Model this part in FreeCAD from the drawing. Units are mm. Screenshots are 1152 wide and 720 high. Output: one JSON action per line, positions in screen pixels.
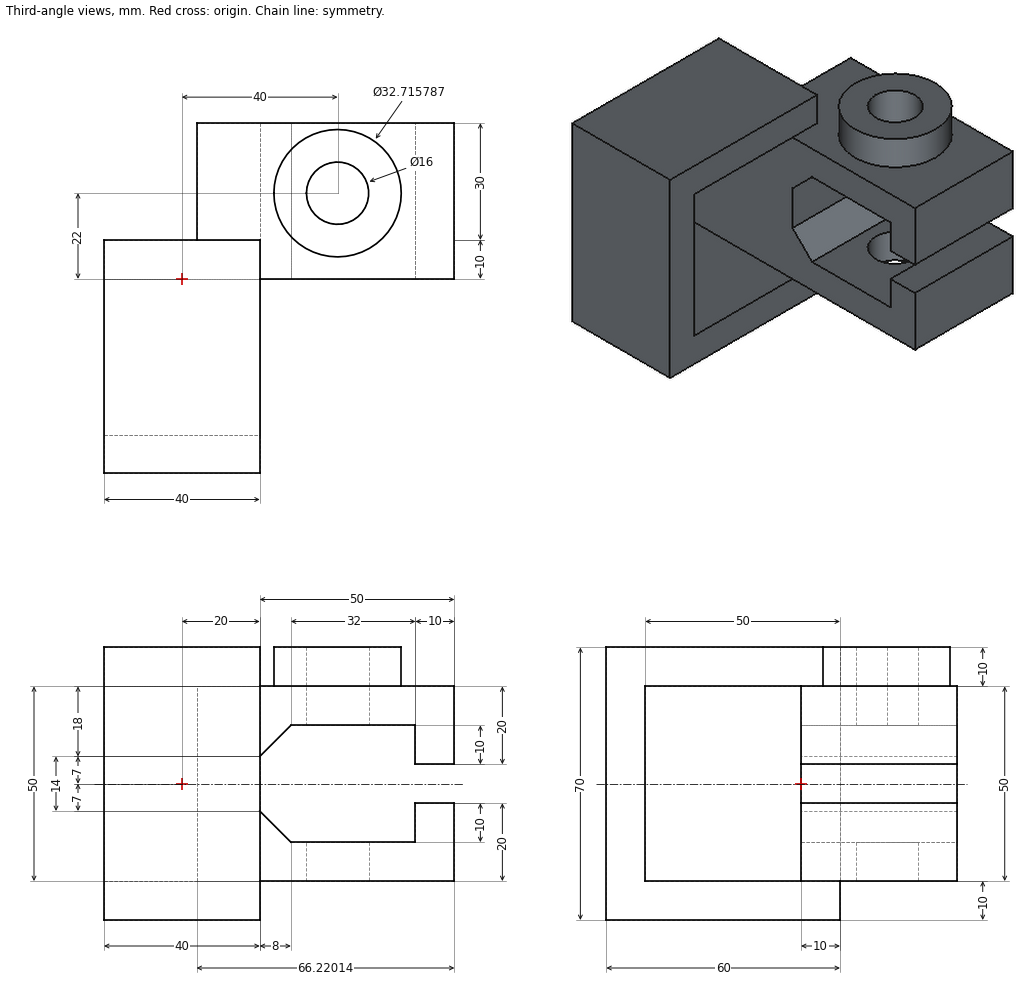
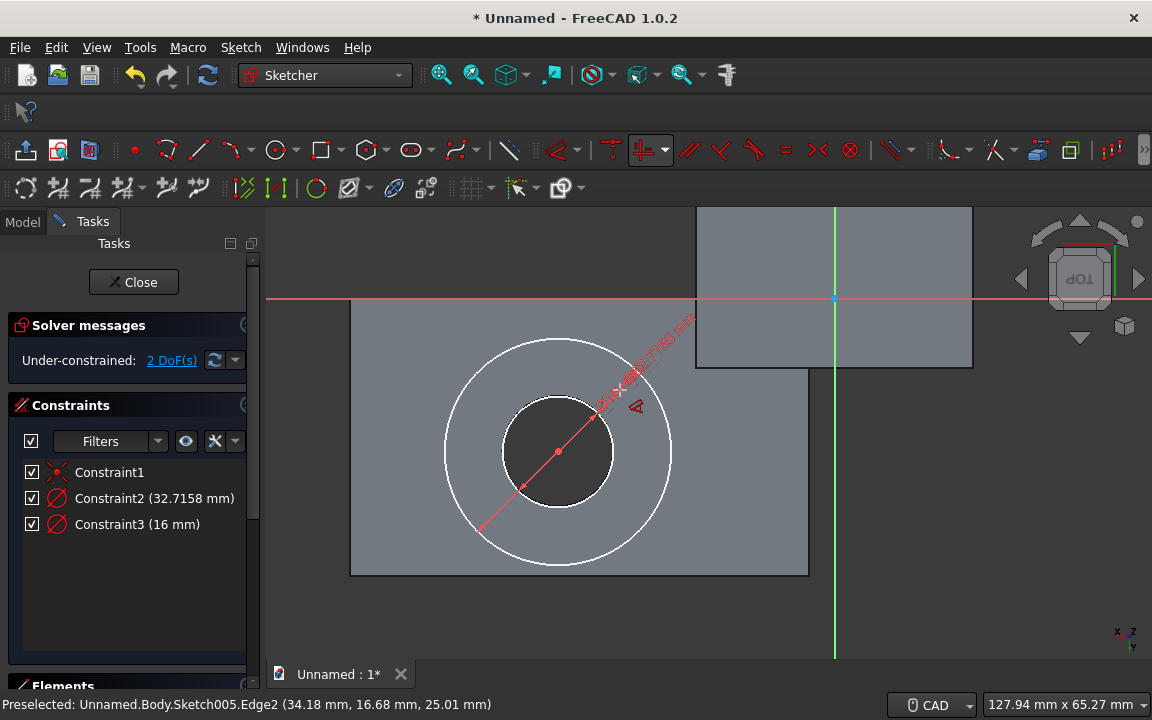
{"action": "left_click", "coordinate": [558, 452]}
{"action": "left_click", "coordinate": [696, 265]}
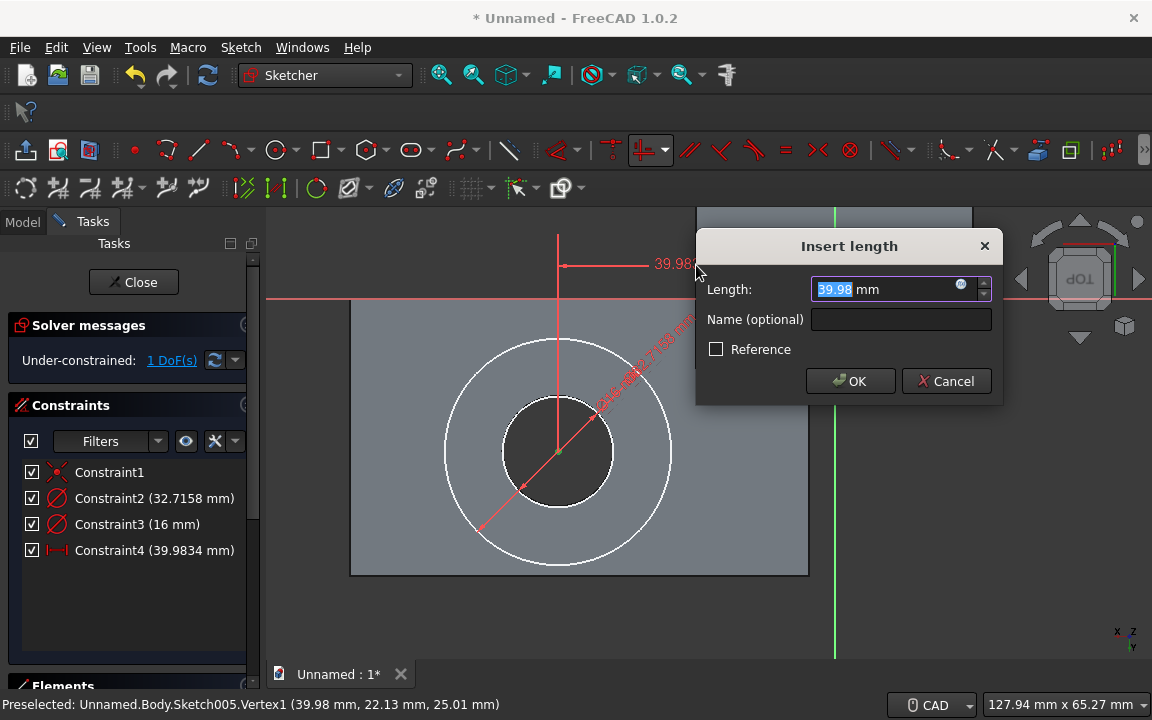
{"action": "type", "text": "40"}
{"action": "key", "text": "Return"}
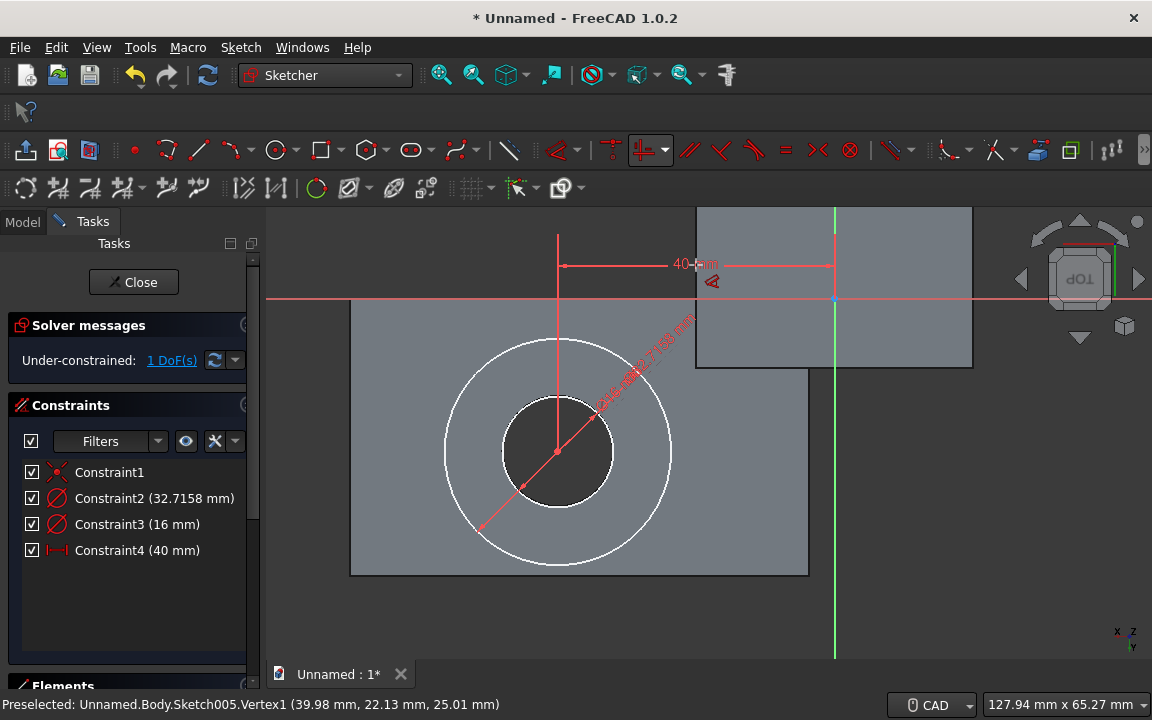
{"action": "left_click", "coordinate": [558, 452]}
{"action": "left_click", "coordinate": [869, 375]}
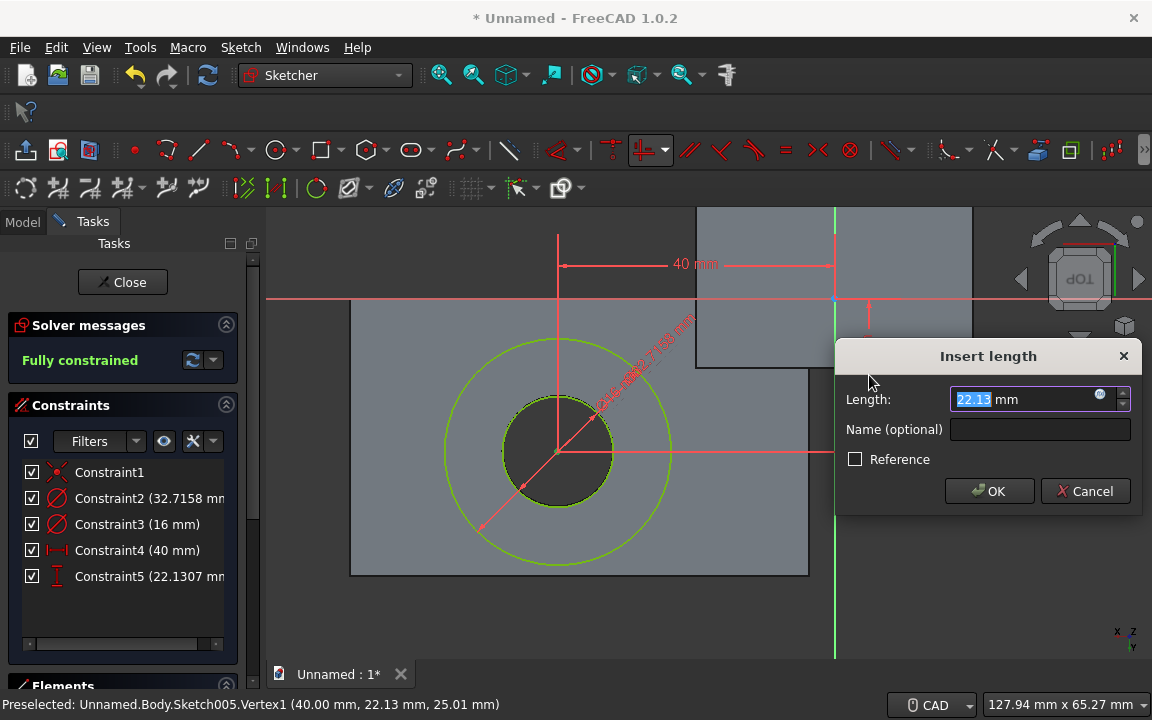
{"action": "type", "text": "22"}
{"action": "key", "text": "Return"}
{"action": "key", "text": "Escape"}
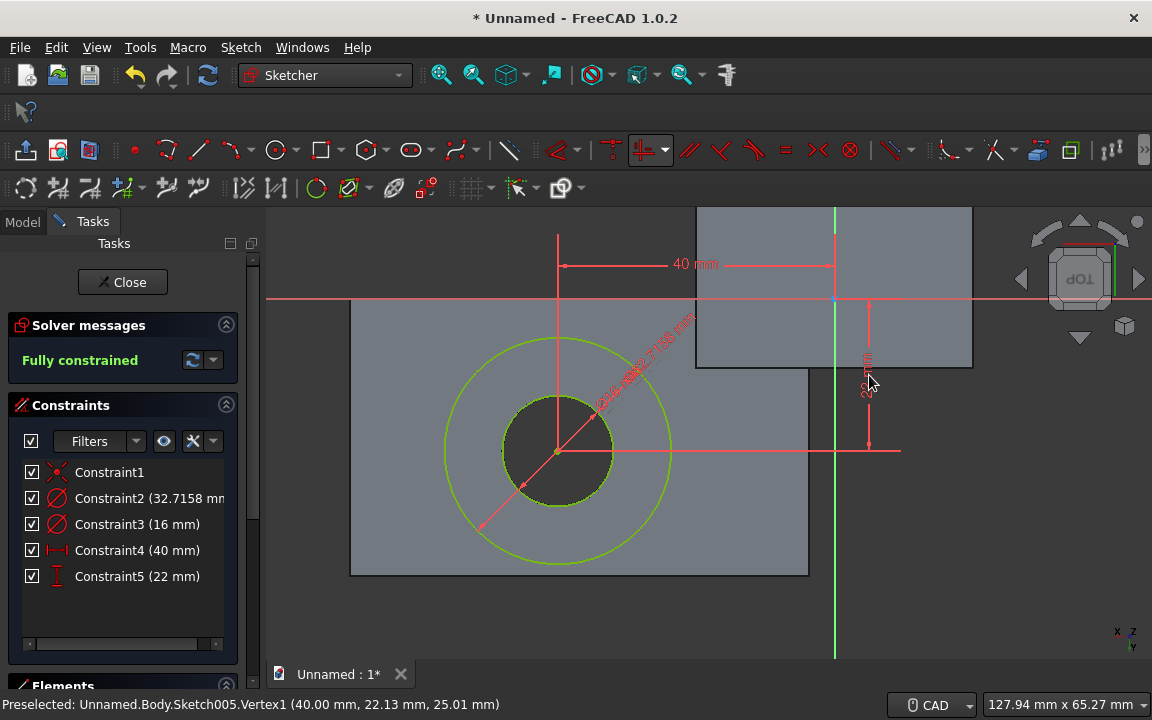
{"action": "left_click", "coordinate": [123, 282]}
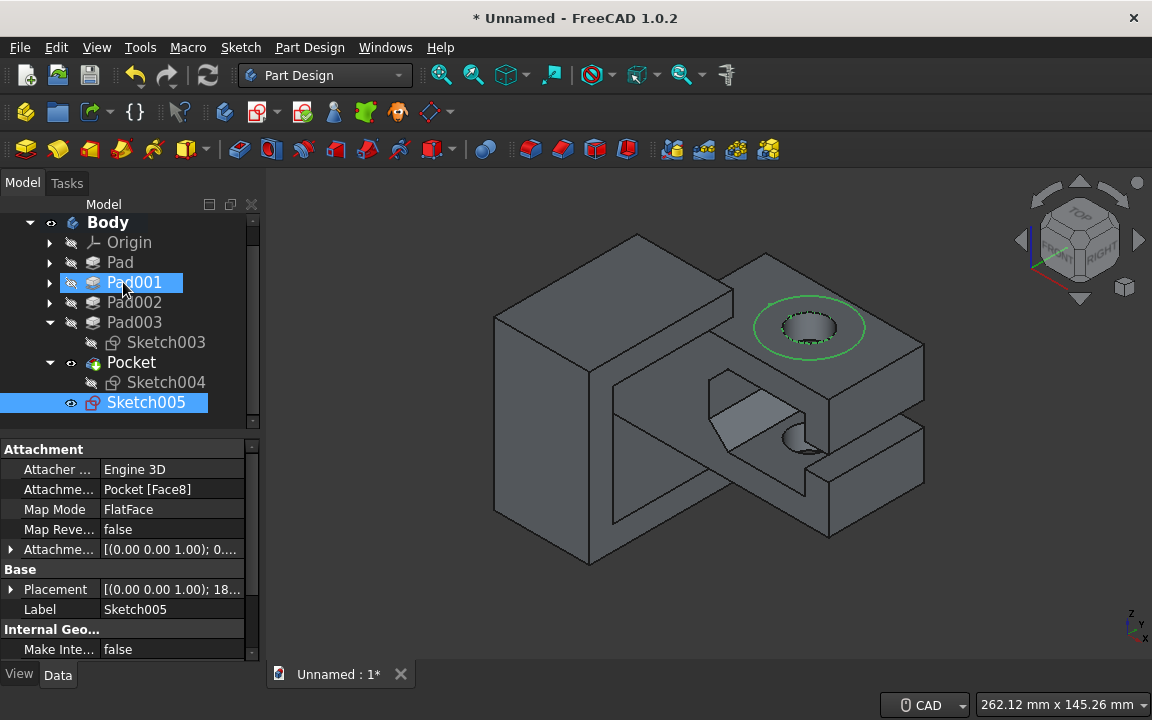
{"action": "left_click", "coordinate": [26, 150]}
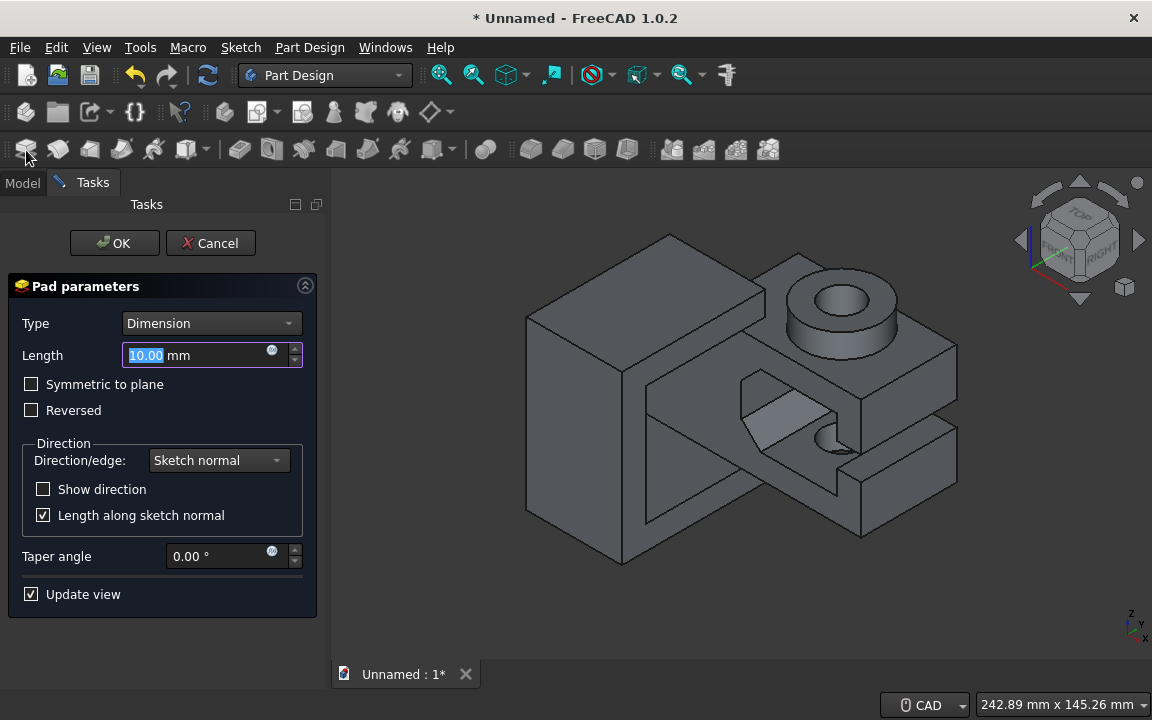
{"action": "type", "text": "10"}
{"action": "key", "text": "Tab"}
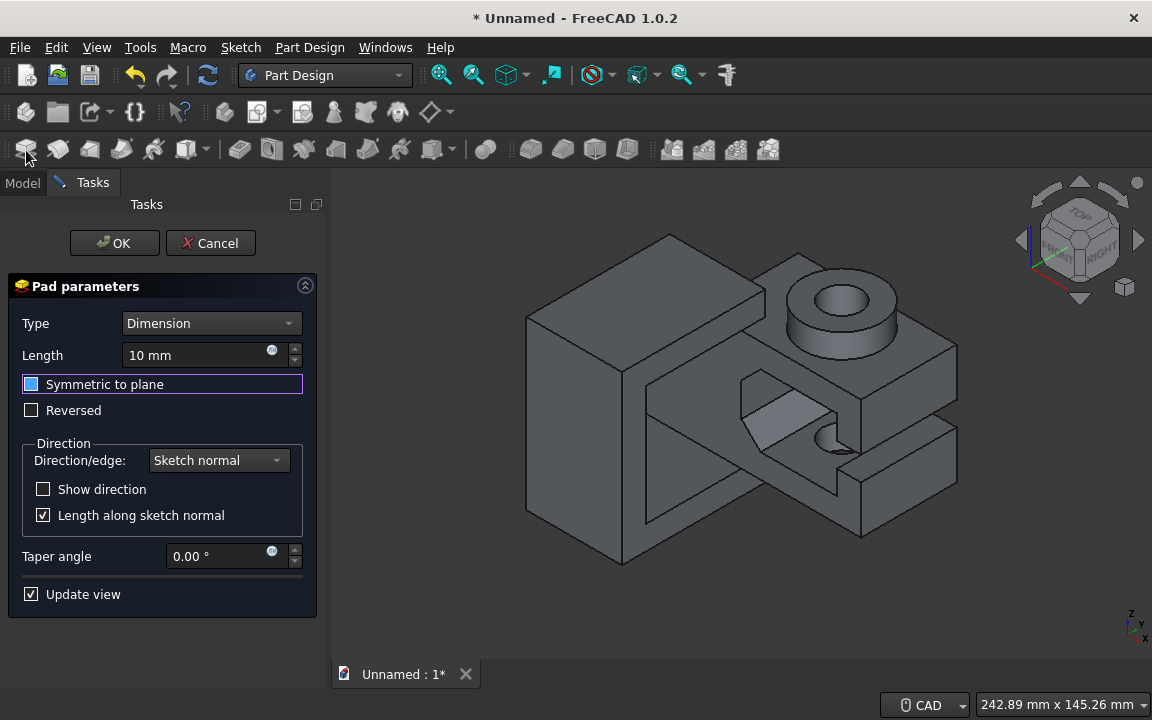
{"action": "left_click", "coordinate": [115, 243]}